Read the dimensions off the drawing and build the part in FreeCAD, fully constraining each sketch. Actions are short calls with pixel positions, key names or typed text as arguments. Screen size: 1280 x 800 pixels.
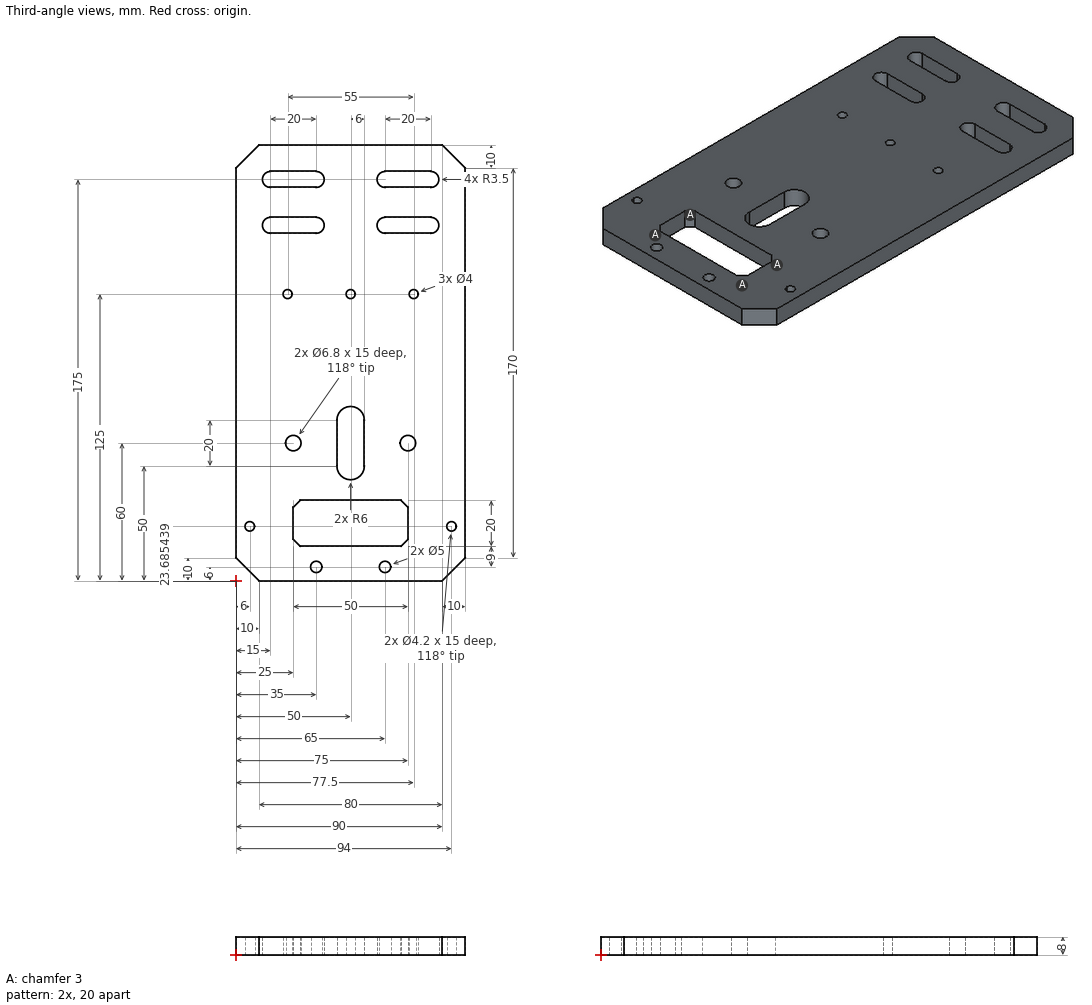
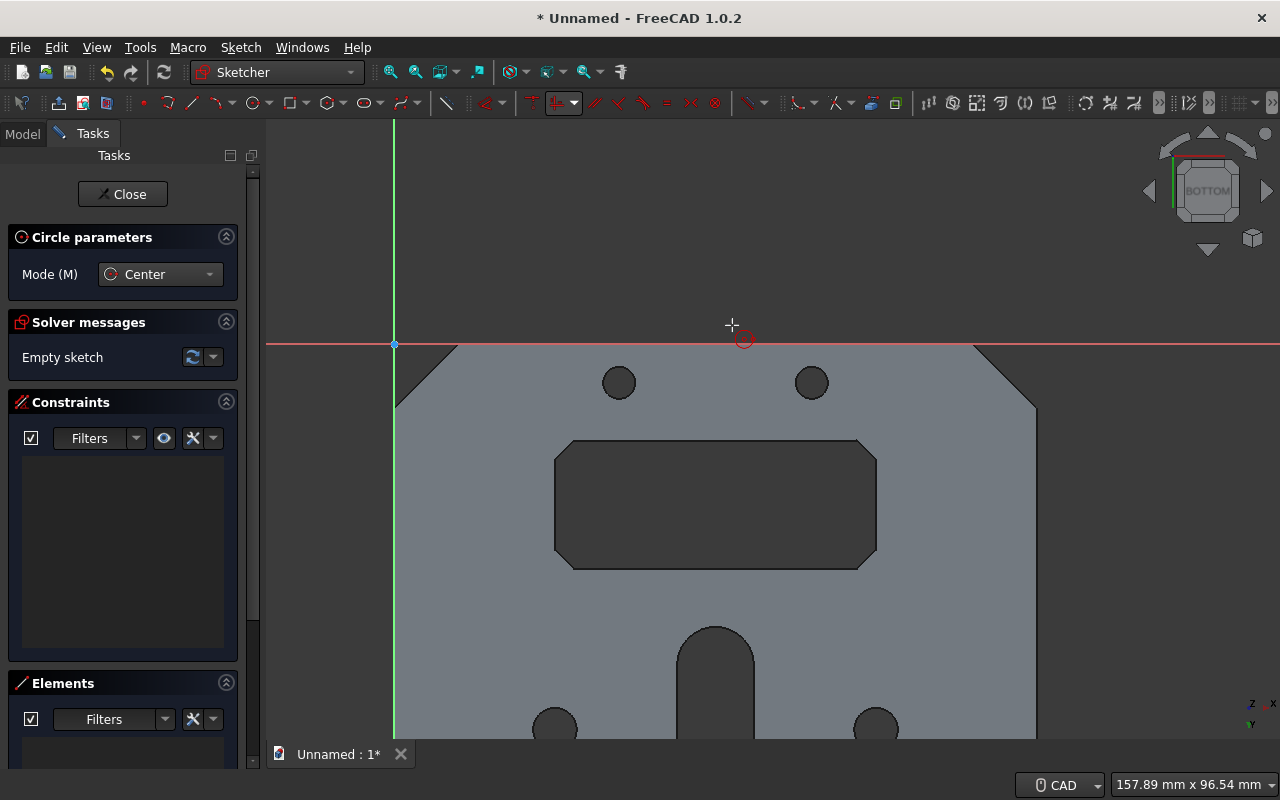
scroll(998, 496, up, 3)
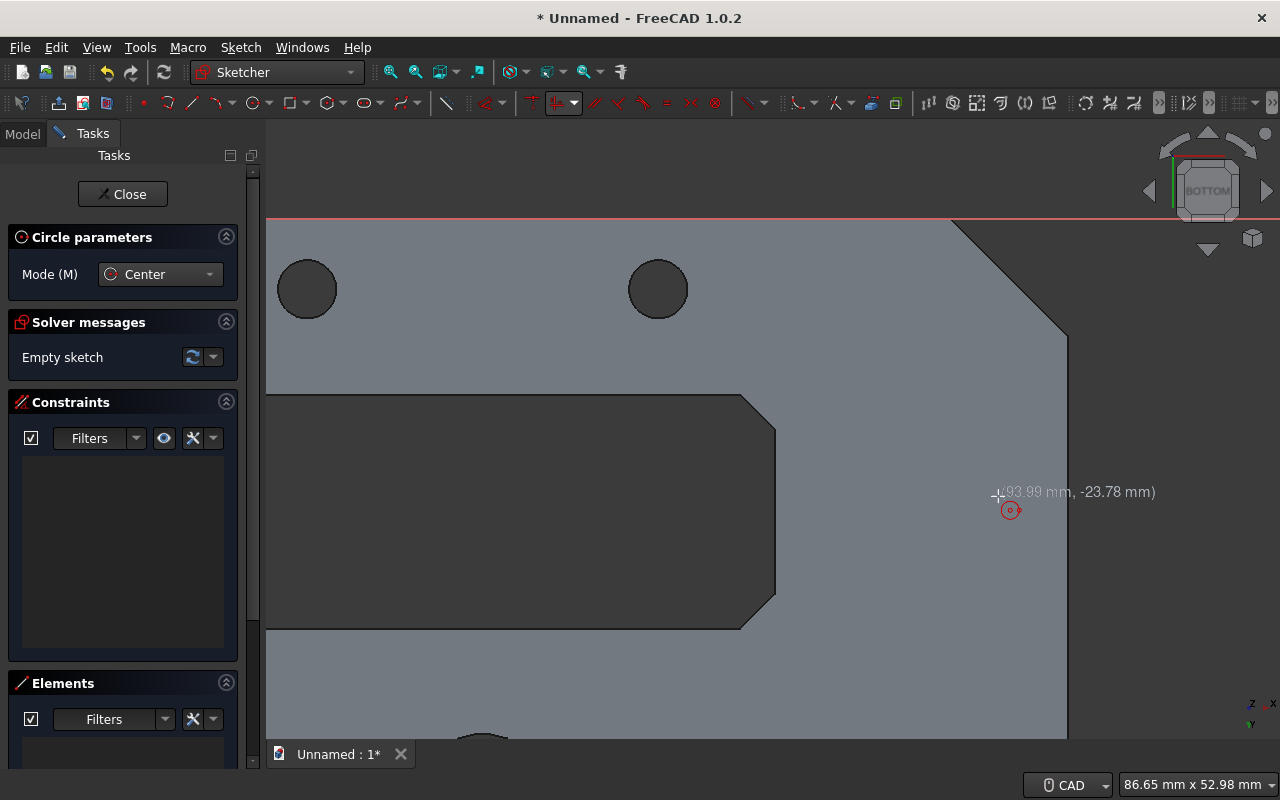
click(998, 496)
move(1015, 479)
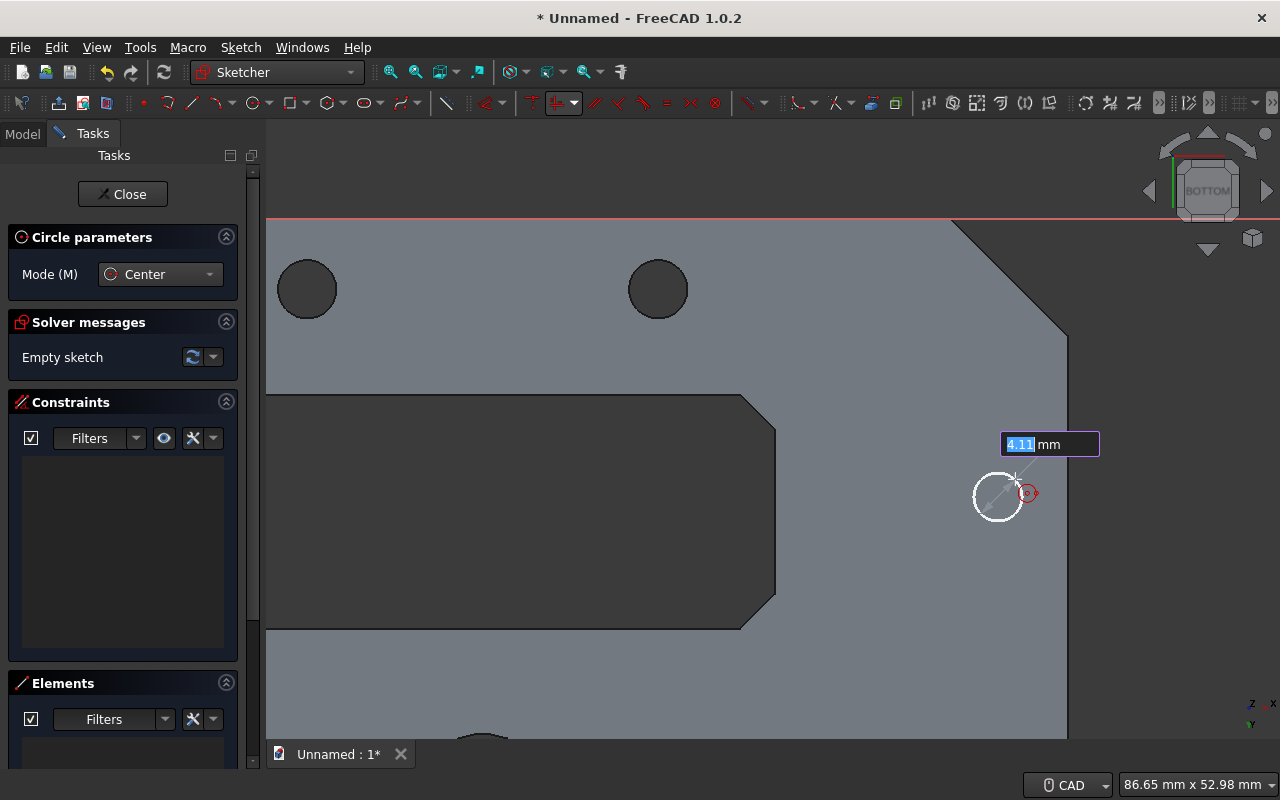
text(4.2)
key(Return)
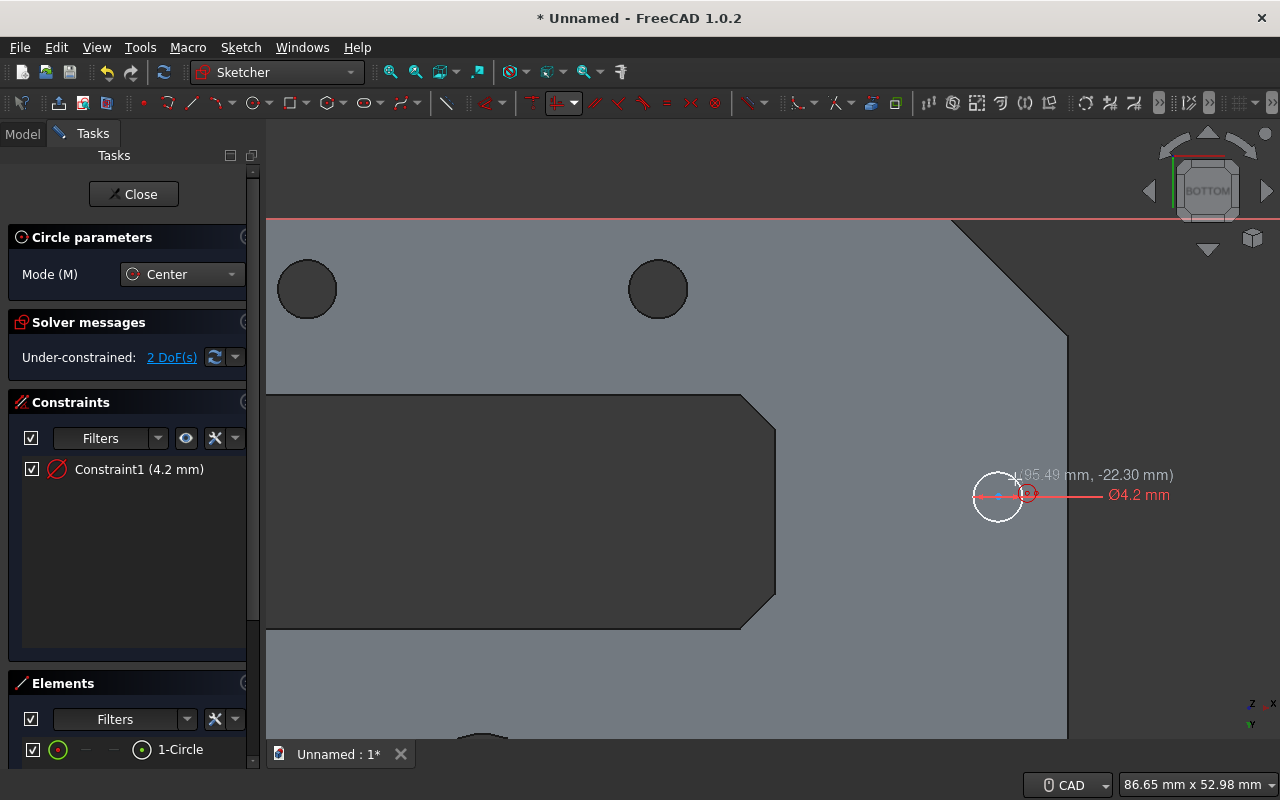
scroll(1002, 501, down, 3)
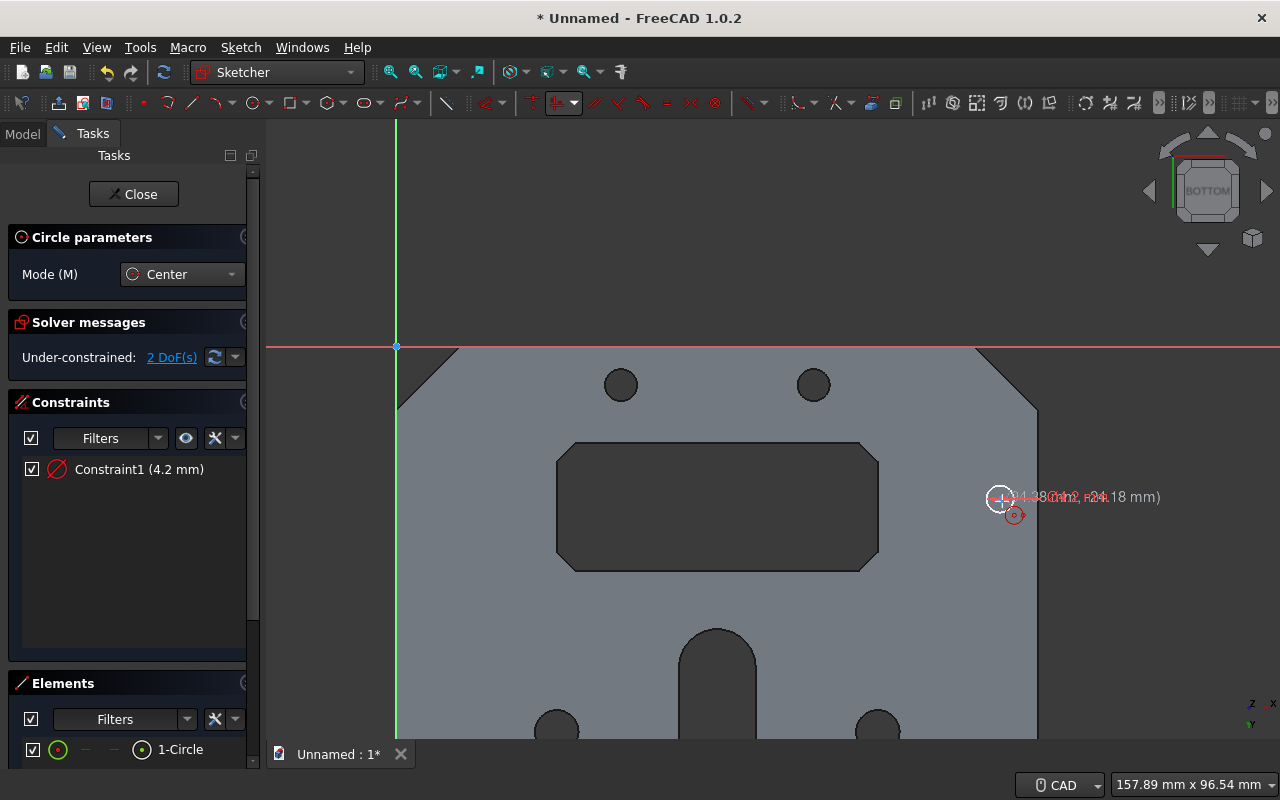
scroll(435, 499, up, 3)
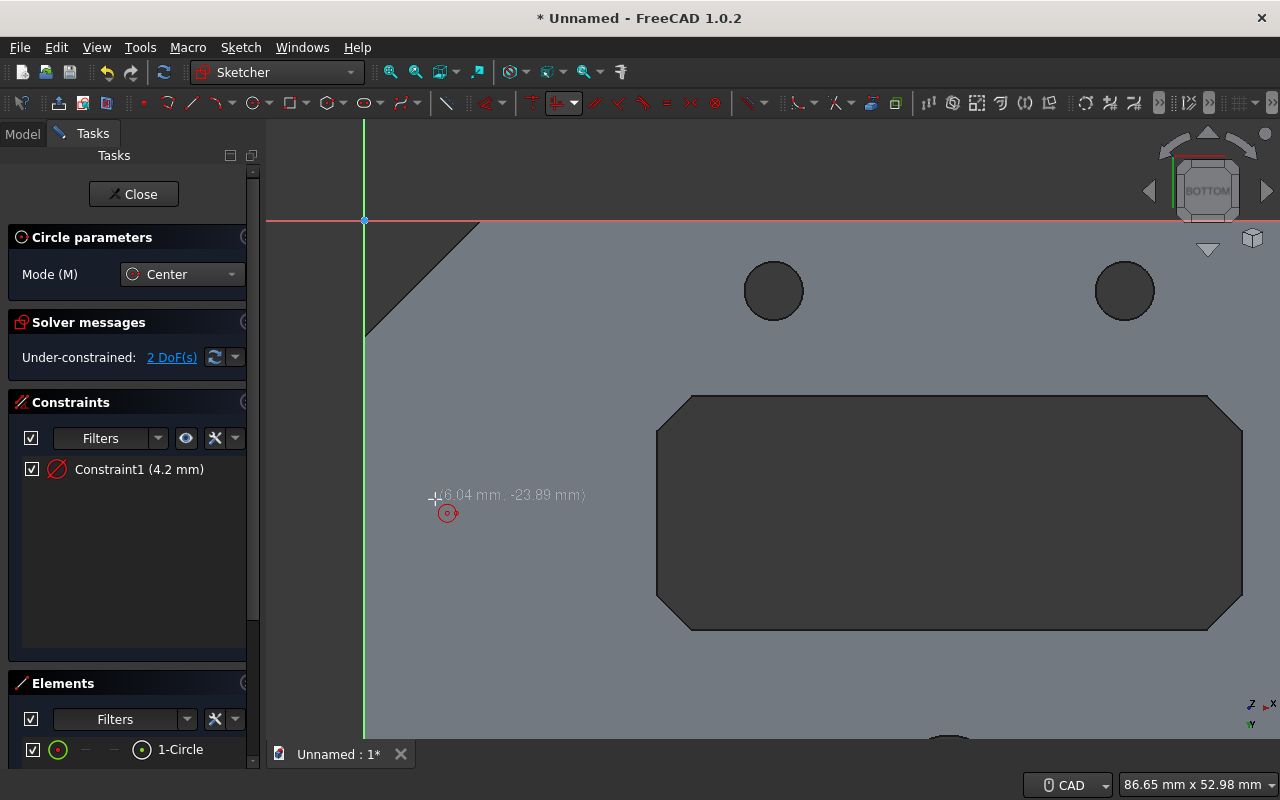
click(434, 498)
move(452, 481)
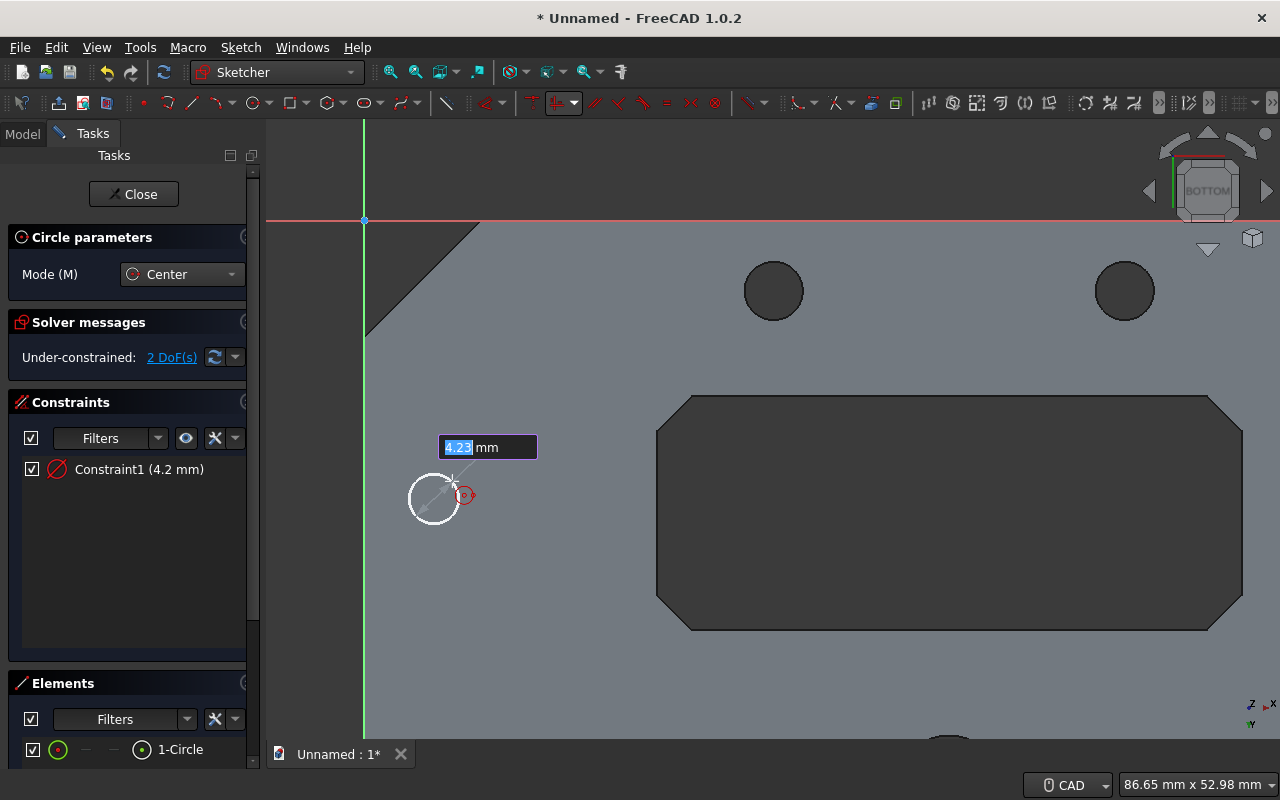
text(4.2)
key(Return)
key(Escape)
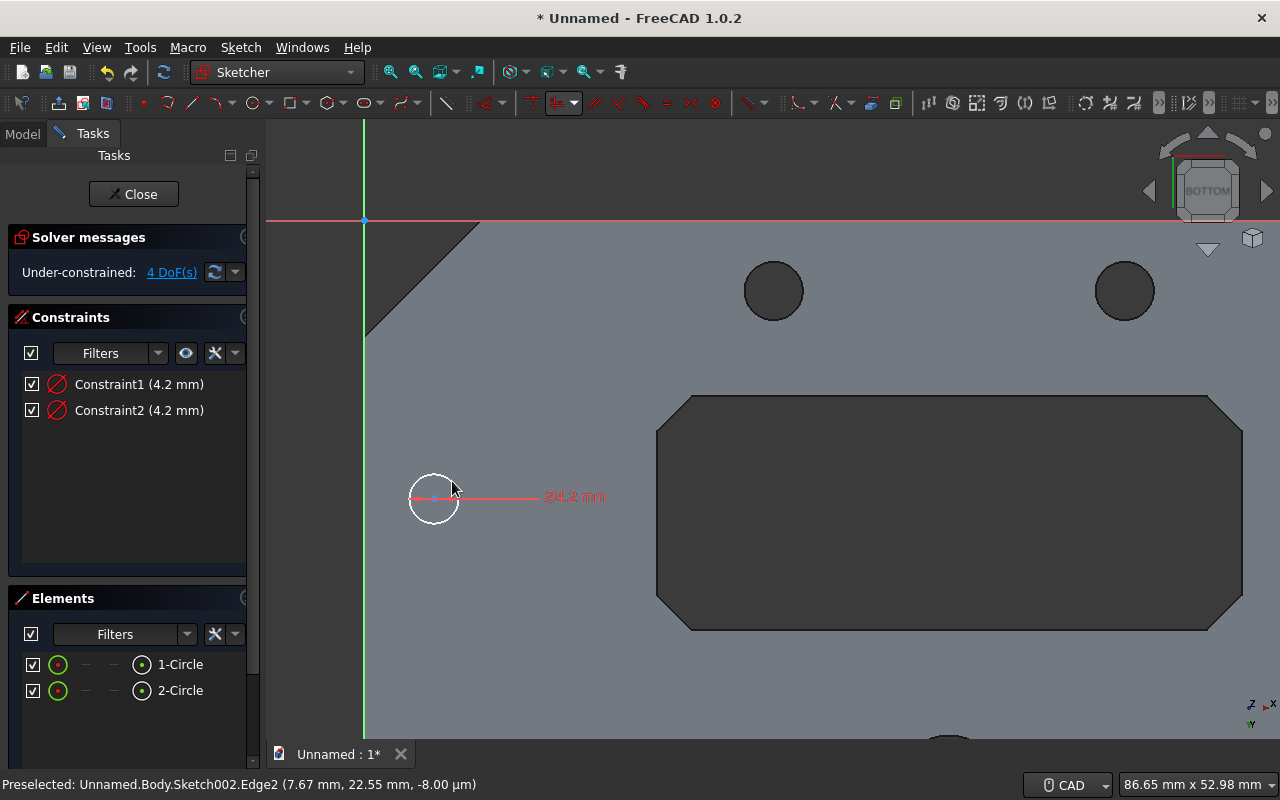
scroll(435, 499, down, 3)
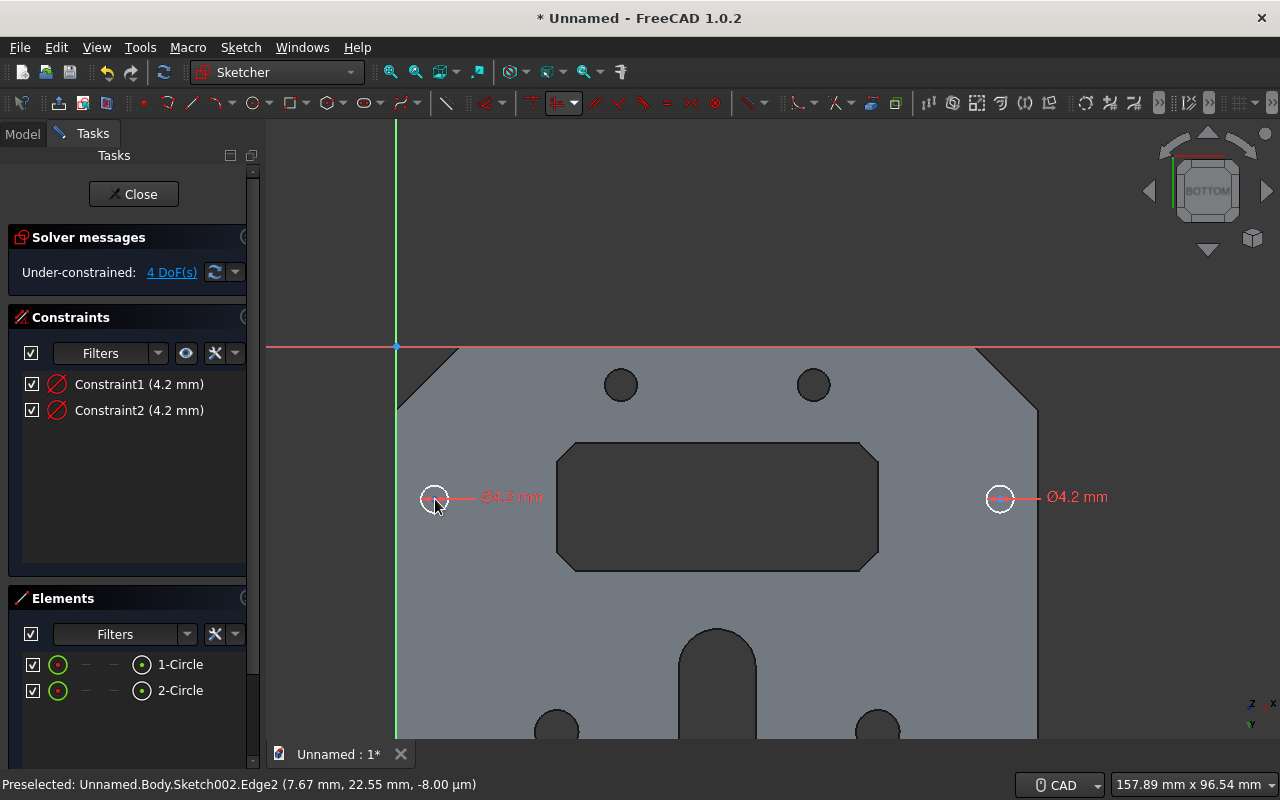
click(1000, 499)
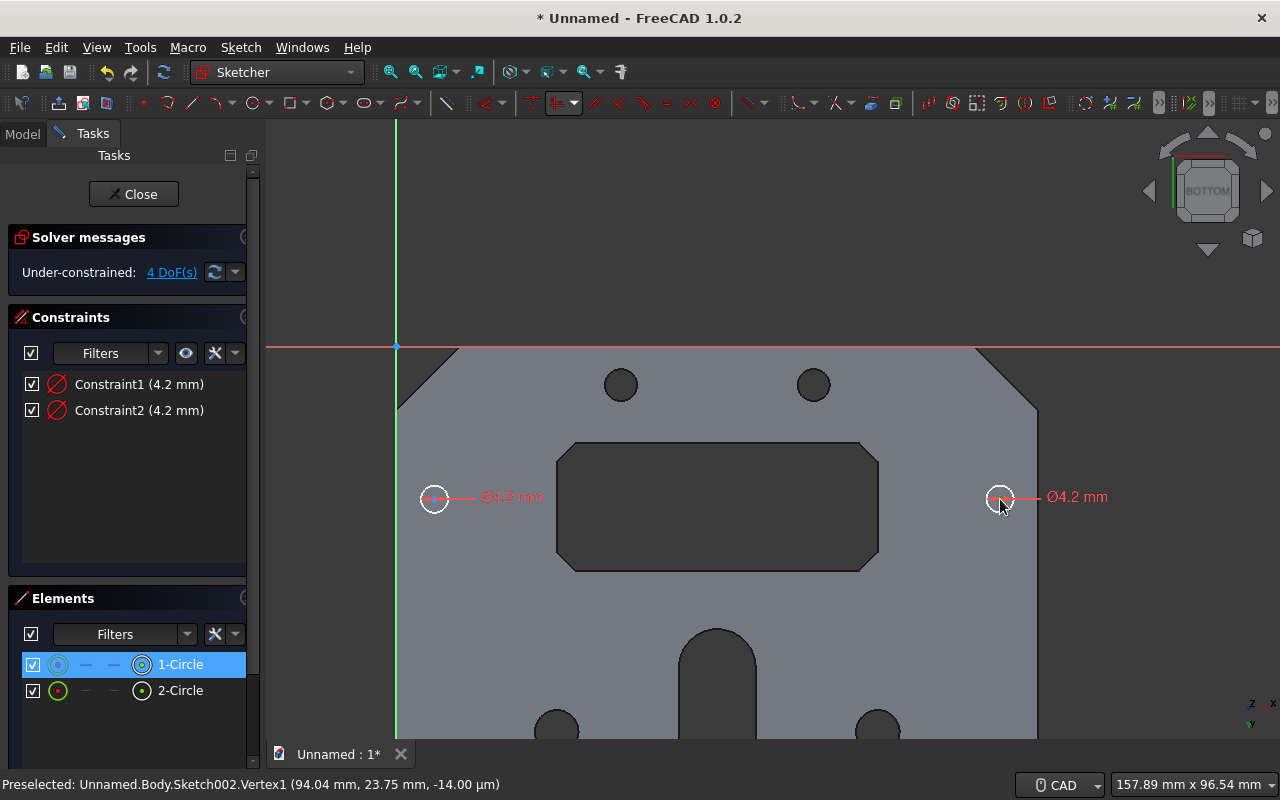
click(435, 499)